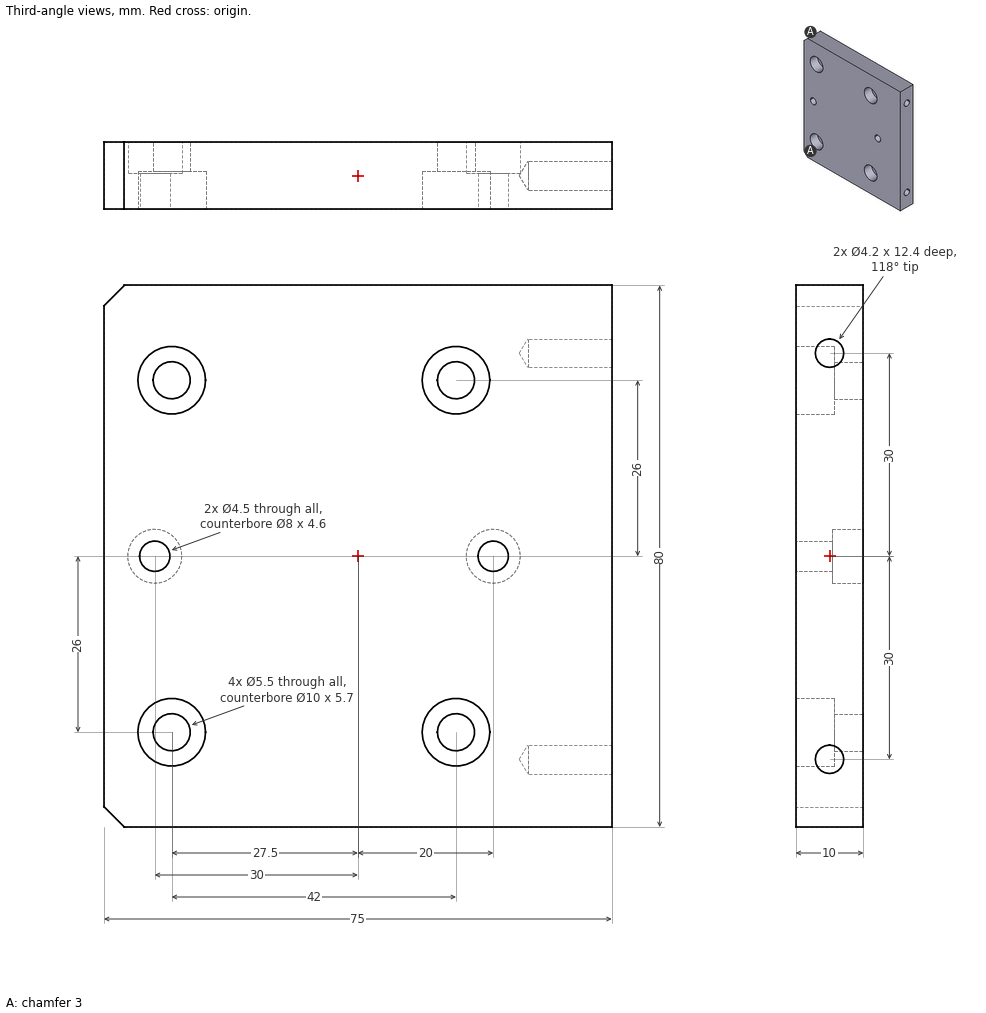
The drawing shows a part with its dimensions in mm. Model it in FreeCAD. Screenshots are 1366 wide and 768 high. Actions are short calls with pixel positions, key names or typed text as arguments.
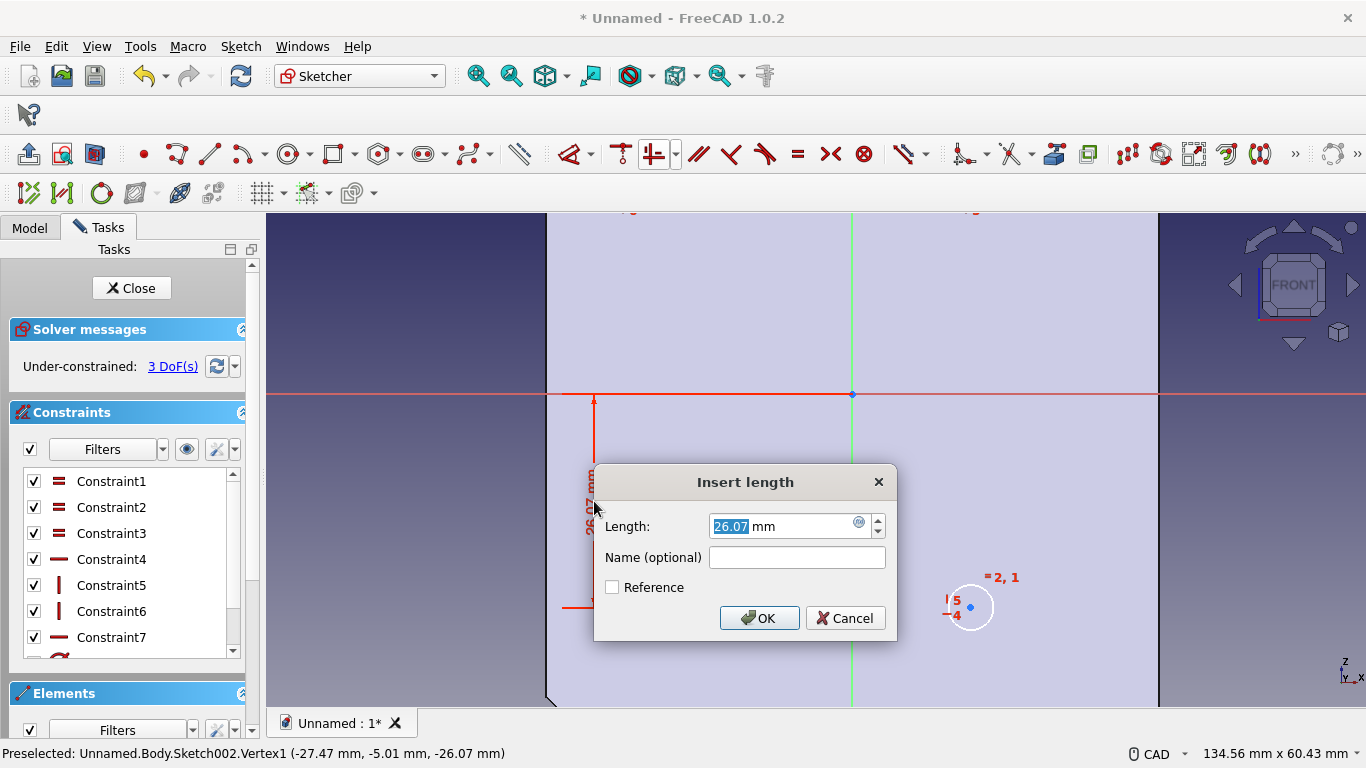
text(26)
key(Return)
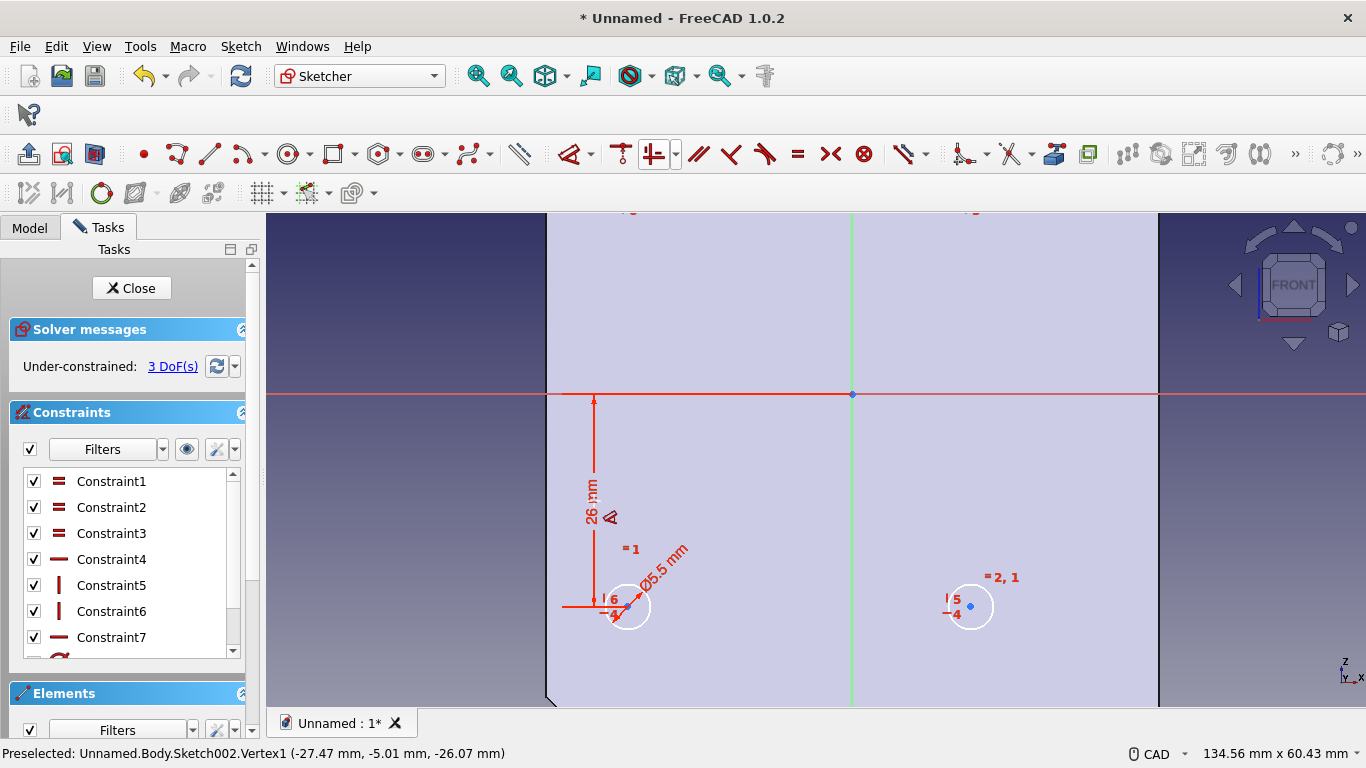
scroll(642, 593, down, 2)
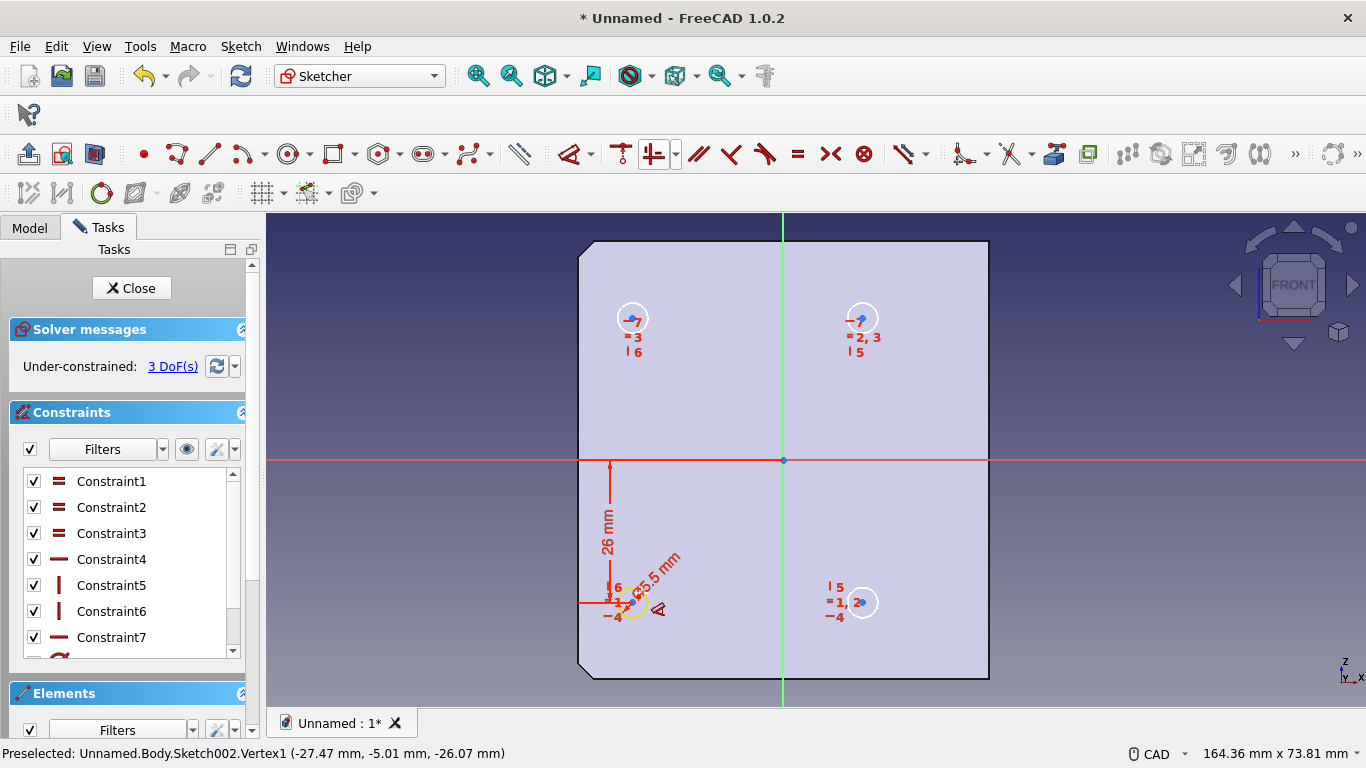
click(863, 318)
click(897, 389)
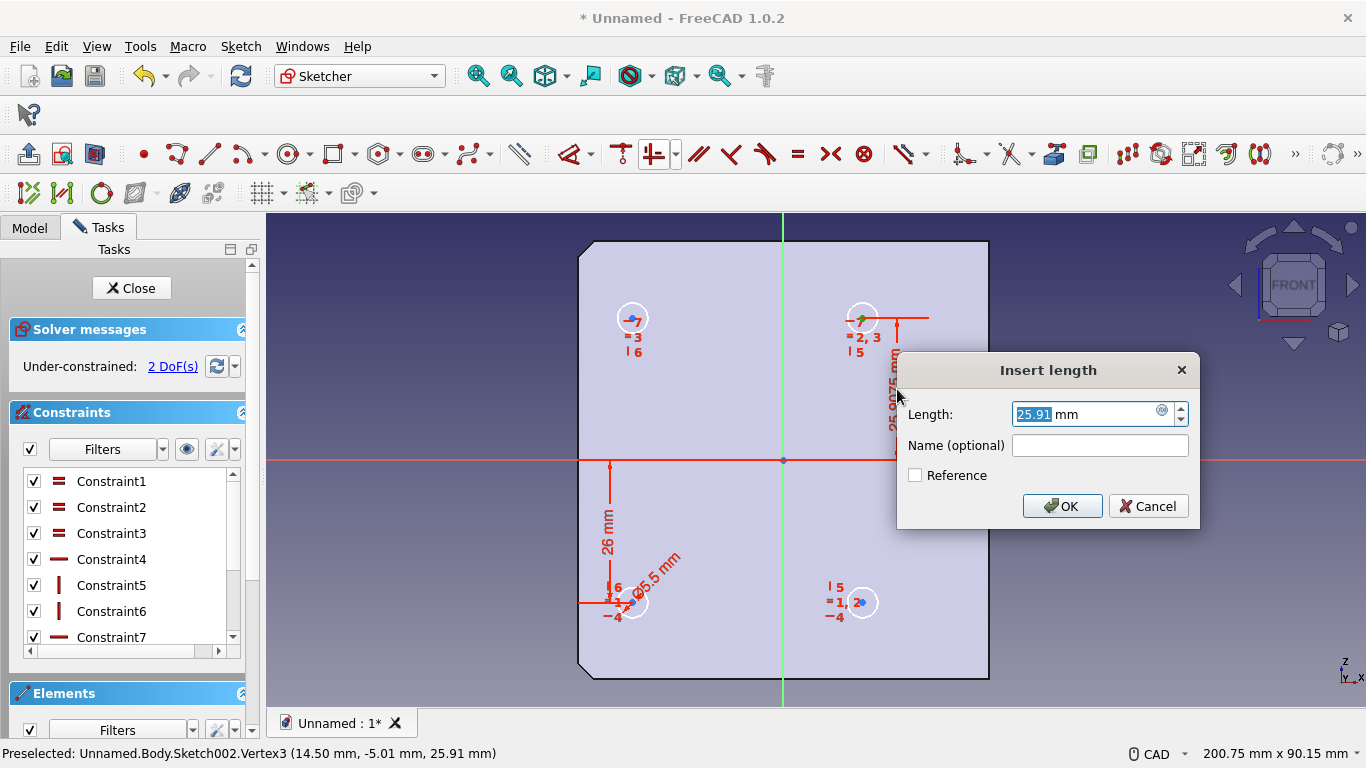
text(26)
key(Return)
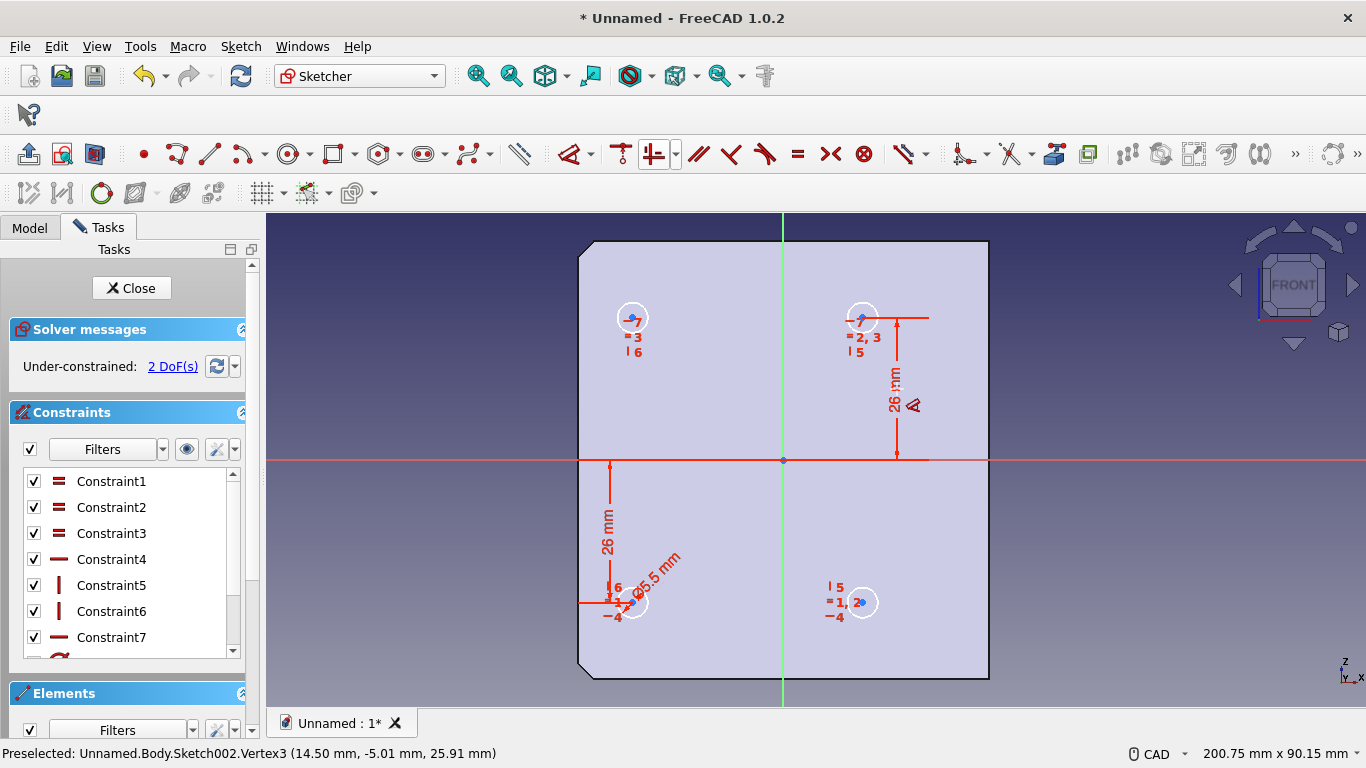
click(633, 603)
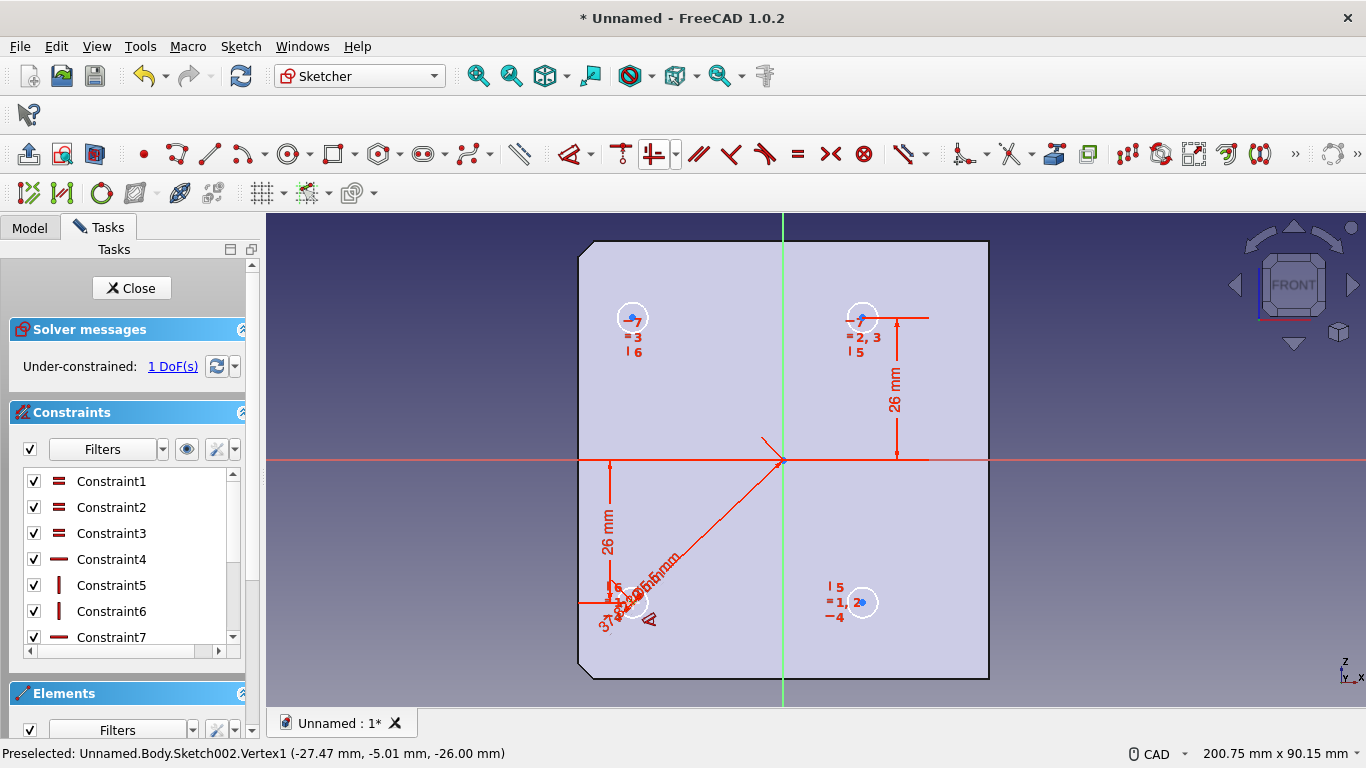
click(863, 603)
click(748, 637)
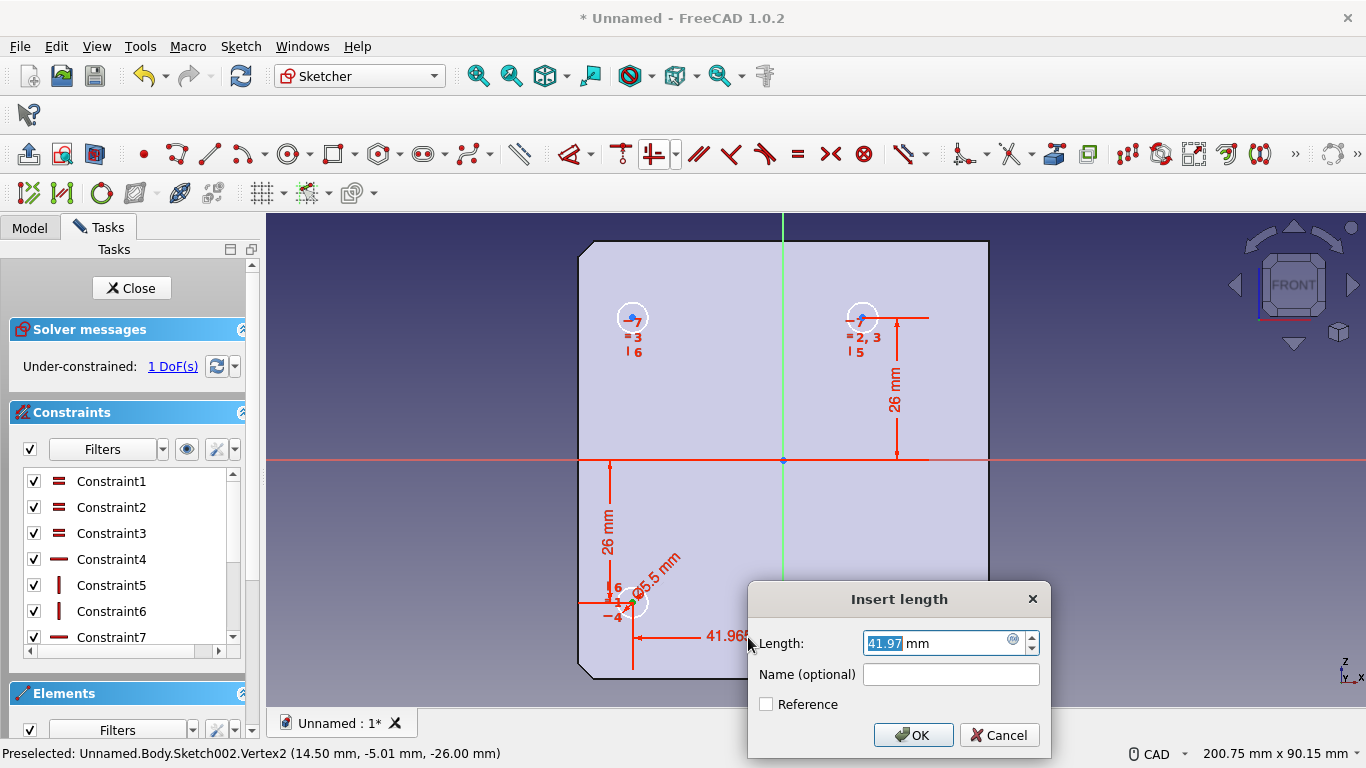
text(42)
key(Return)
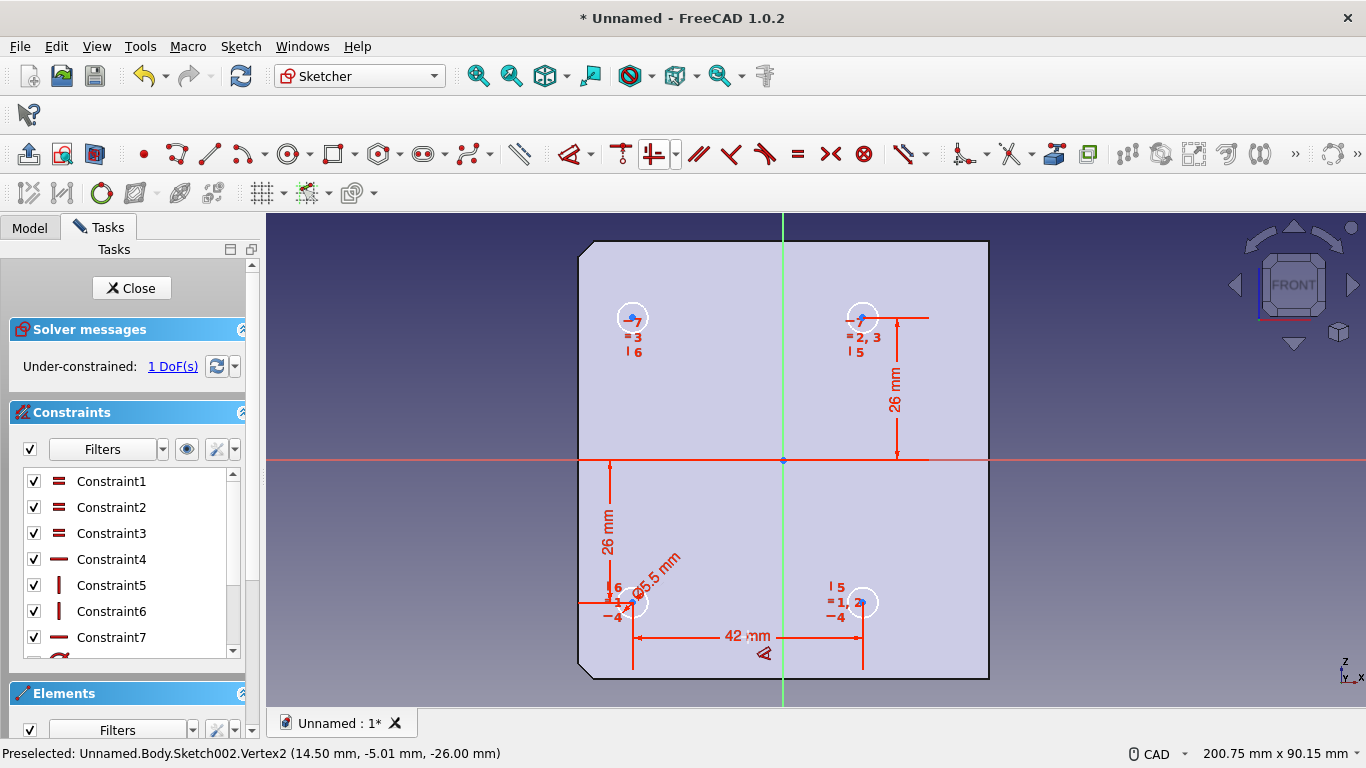
click(633, 603)
click(673, 637)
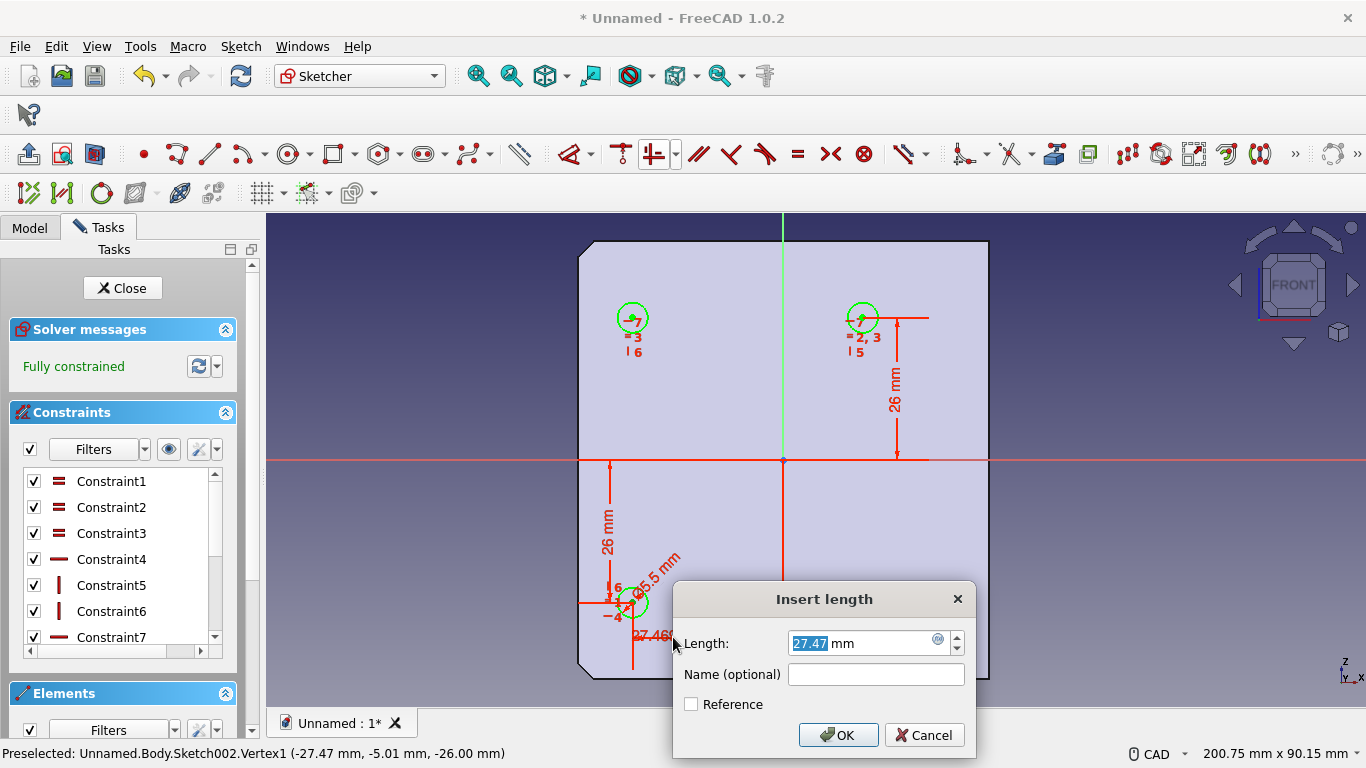
text(27.5)
key(Return)
key(Escape)